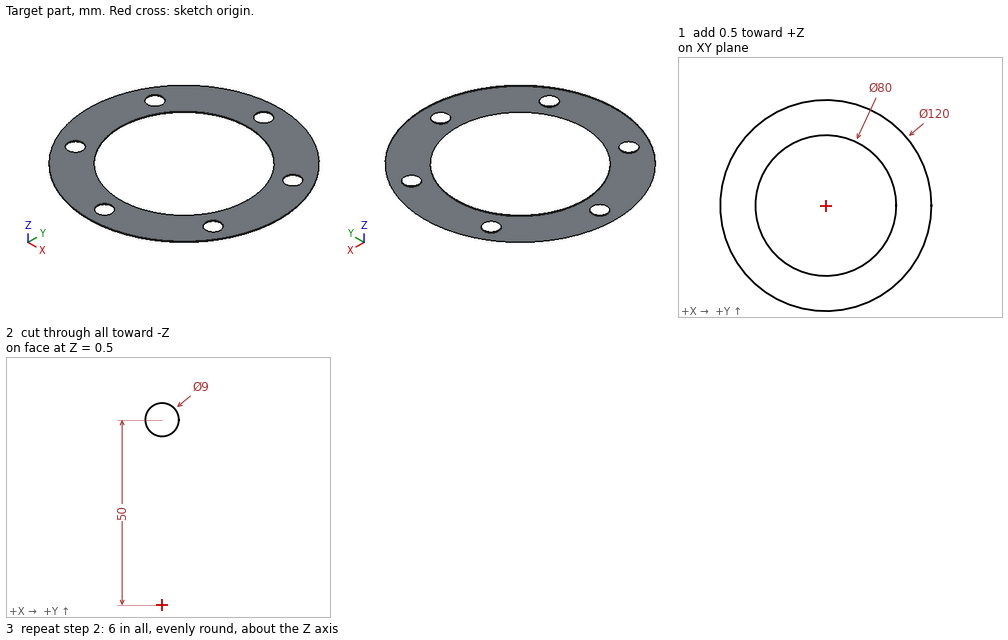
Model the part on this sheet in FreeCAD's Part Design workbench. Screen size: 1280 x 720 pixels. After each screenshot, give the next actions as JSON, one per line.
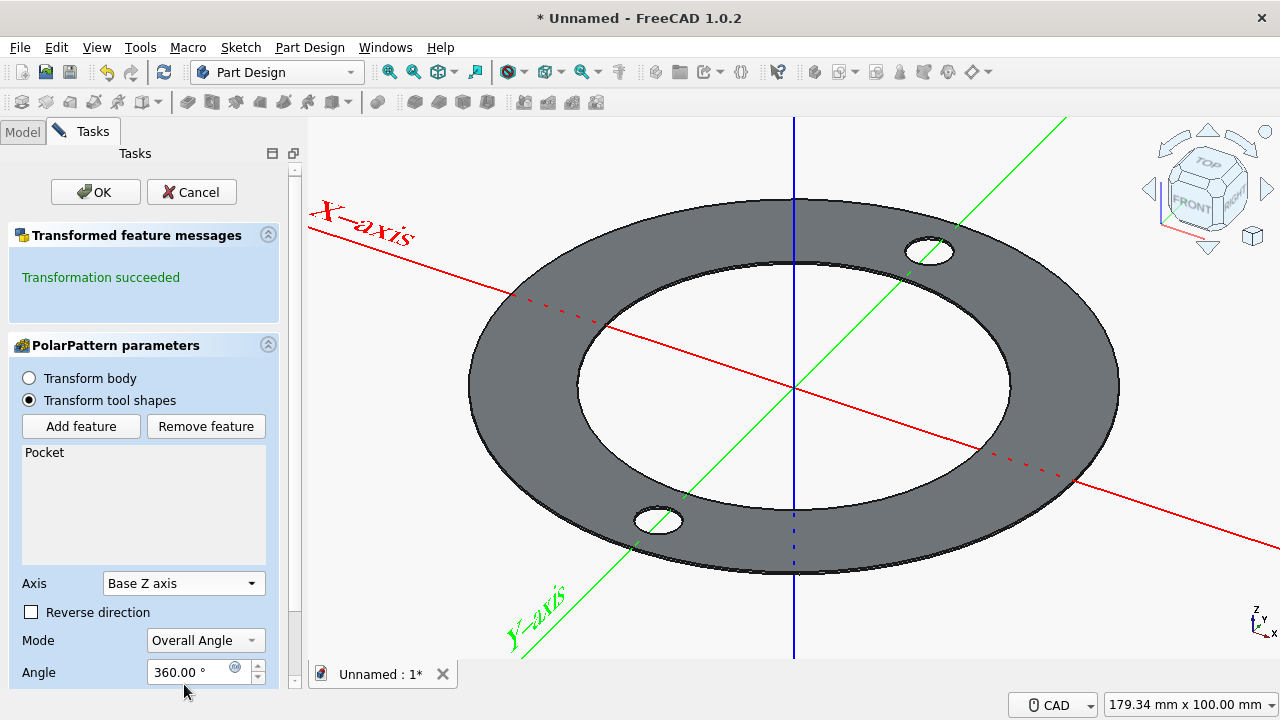
{"action": "scroll", "coordinate": [295, 426], "scroll_direction": "down", "scroll_amount": 2}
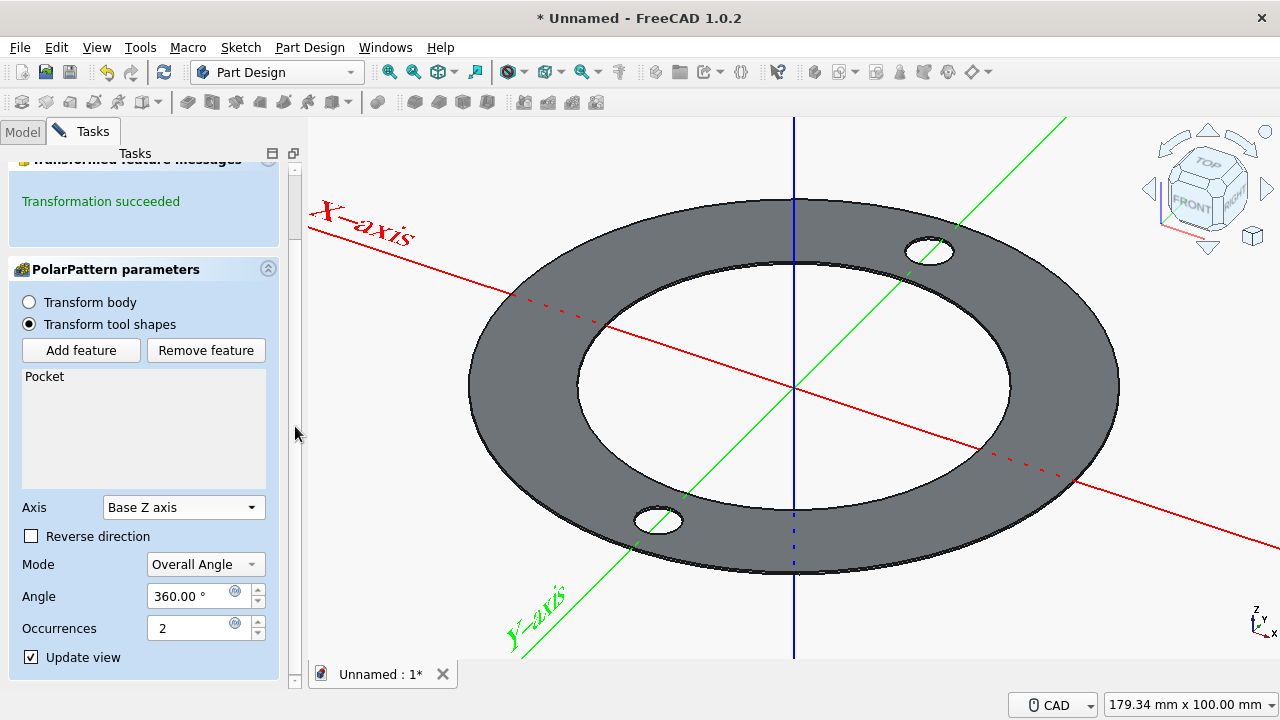
{"action": "triple_click", "coordinate": [198, 628]}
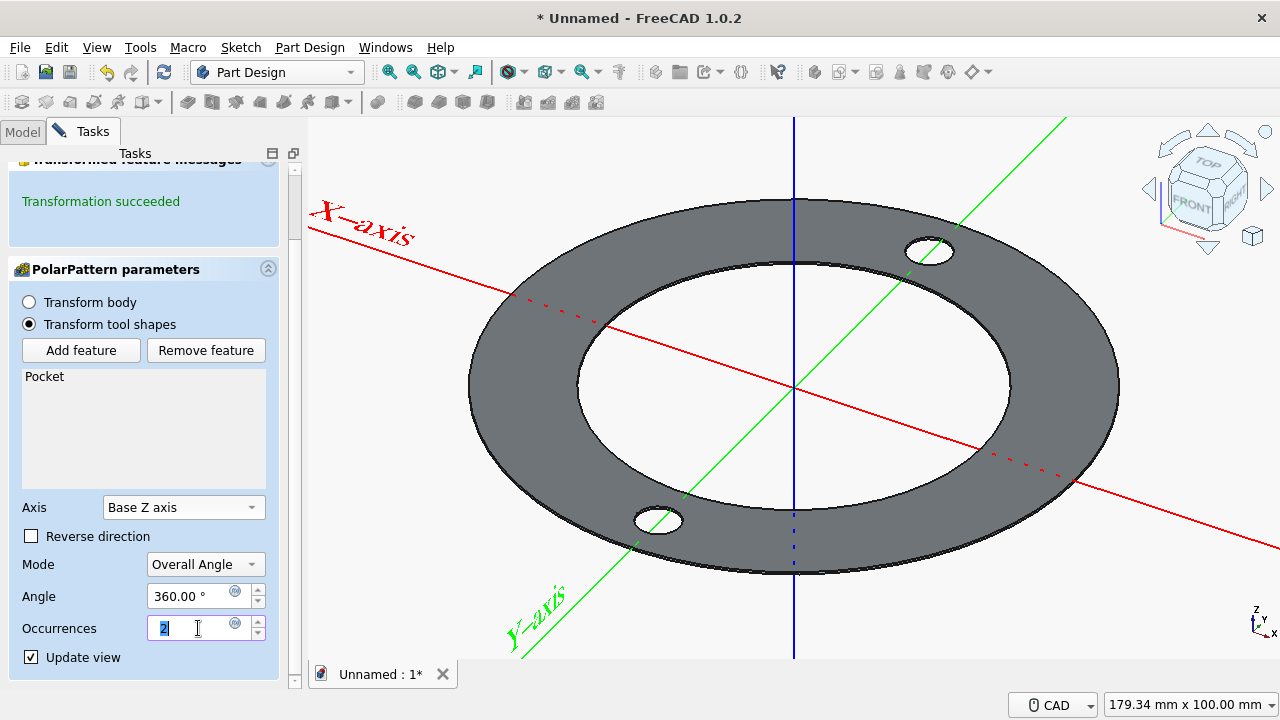
{"action": "type", "text": "6"}
{"action": "key", "text": "Tab"}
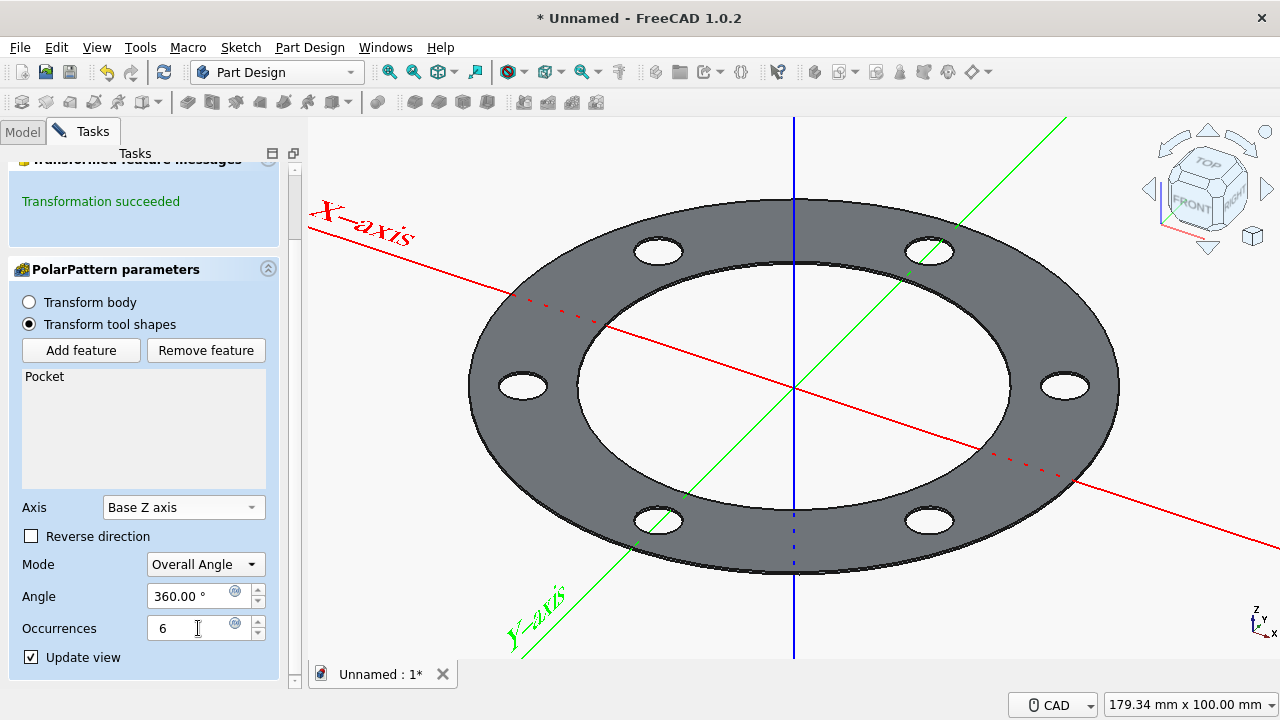
{"action": "scroll", "coordinate": [295, 426], "scroll_direction": "up", "scroll_amount": 3}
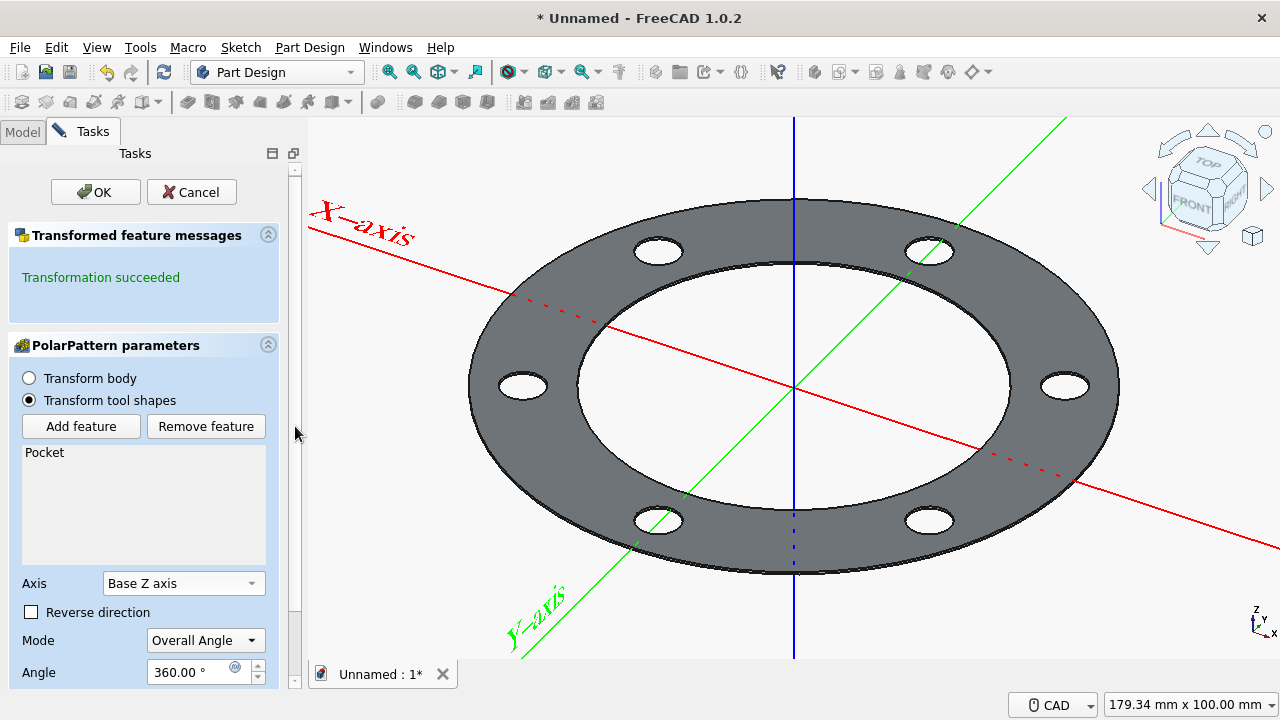
{"action": "left_click", "coordinate": [96, 192]}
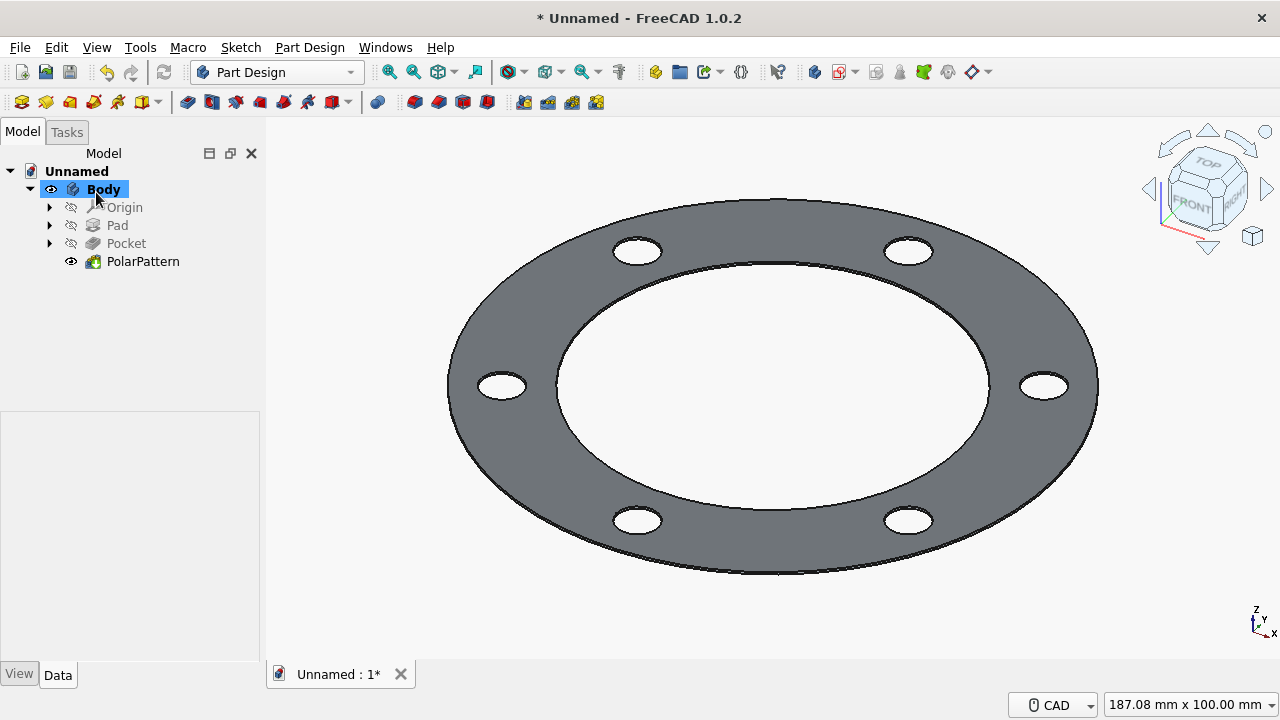
{"action": "key", "text": "0"}